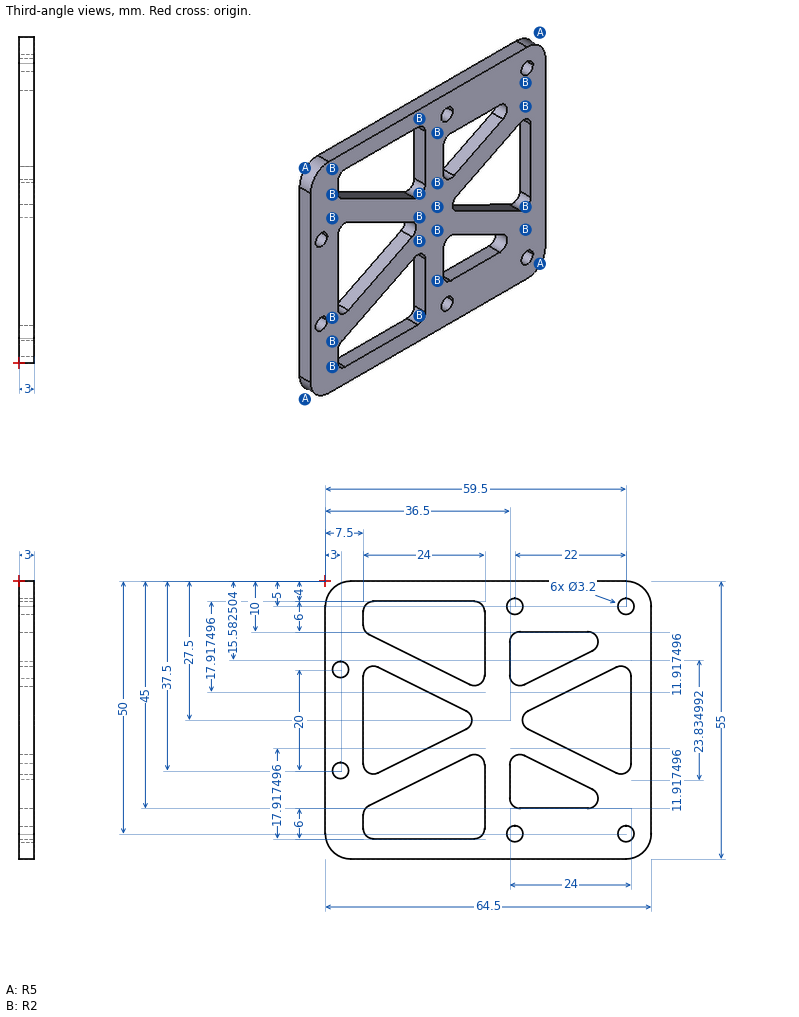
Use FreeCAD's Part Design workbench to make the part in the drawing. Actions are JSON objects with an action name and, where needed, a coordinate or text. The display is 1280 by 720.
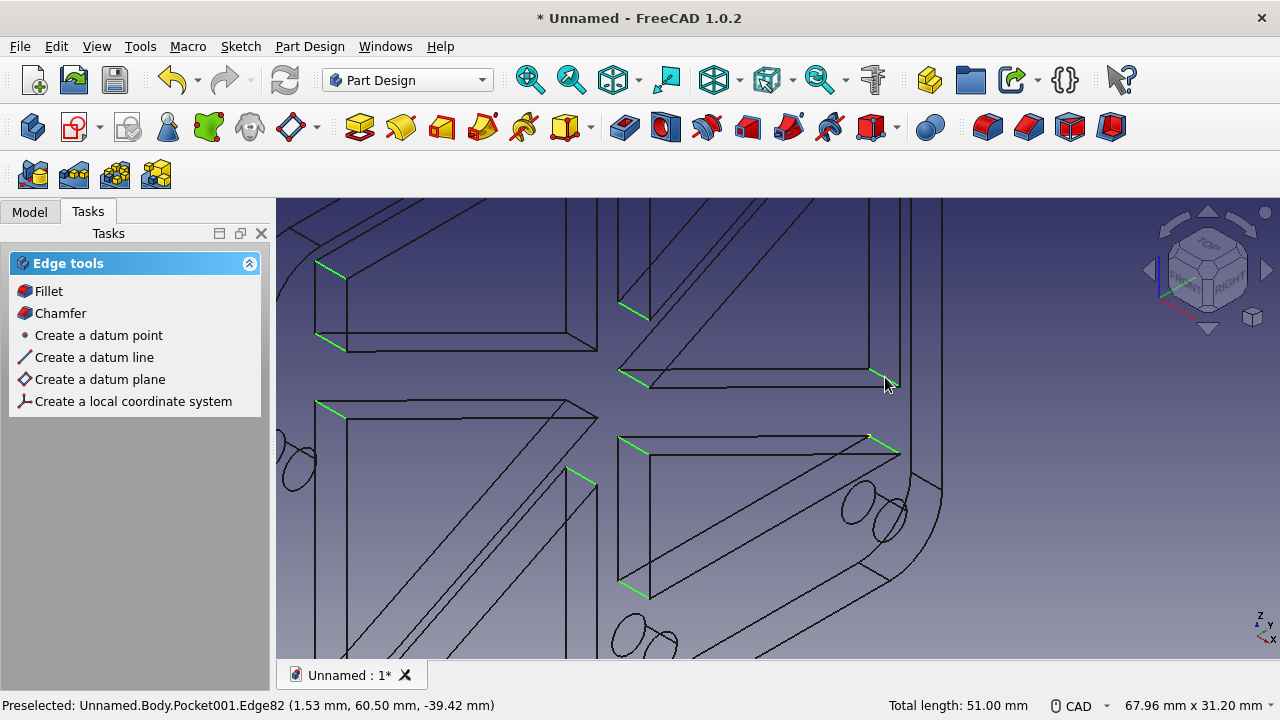
{"action": "left_click", "coordinate": [582, 408], "text": "ctrl"}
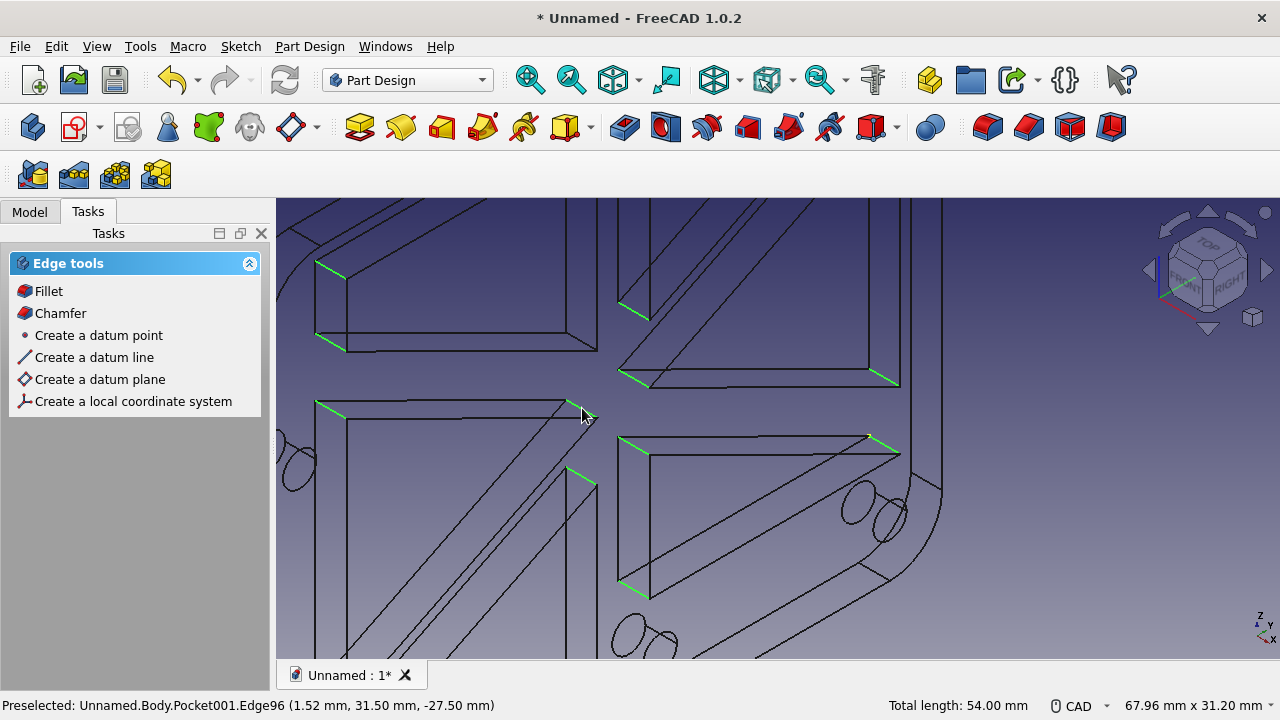
{"action": "left_click", "coordinate": [582, 341], "text": "ctrl"}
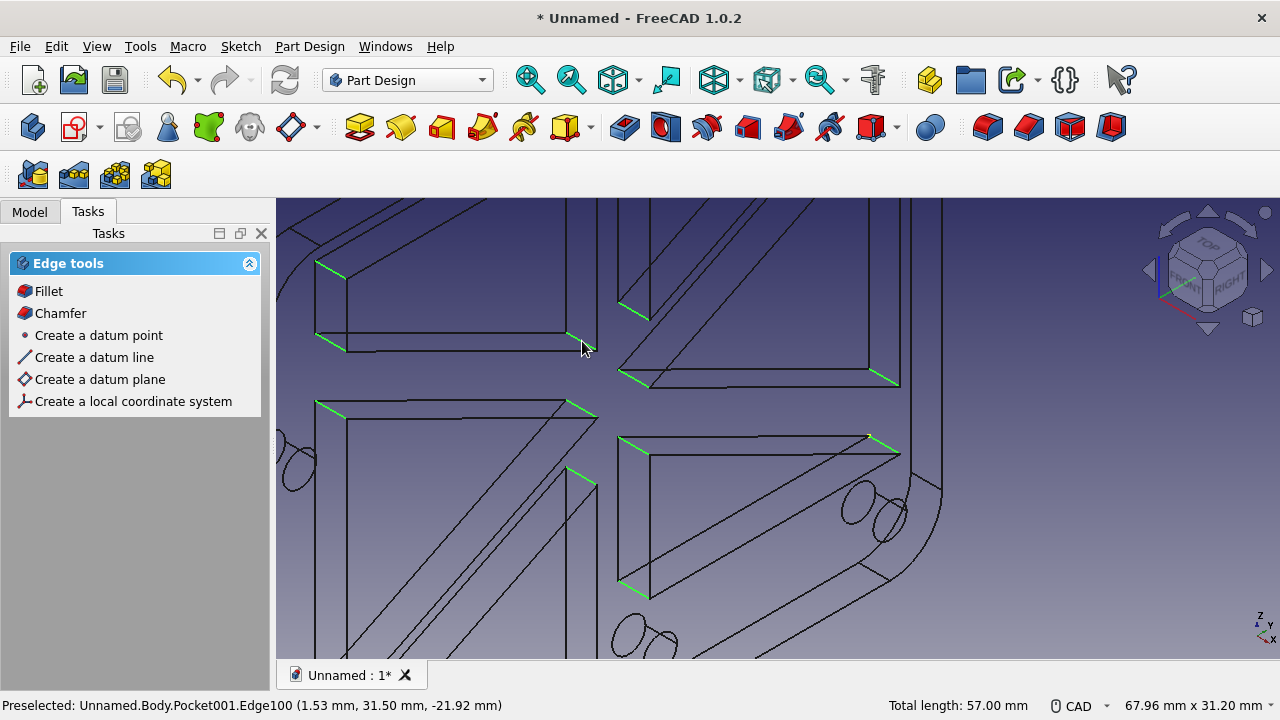
{"action": "key", "text": "v f"}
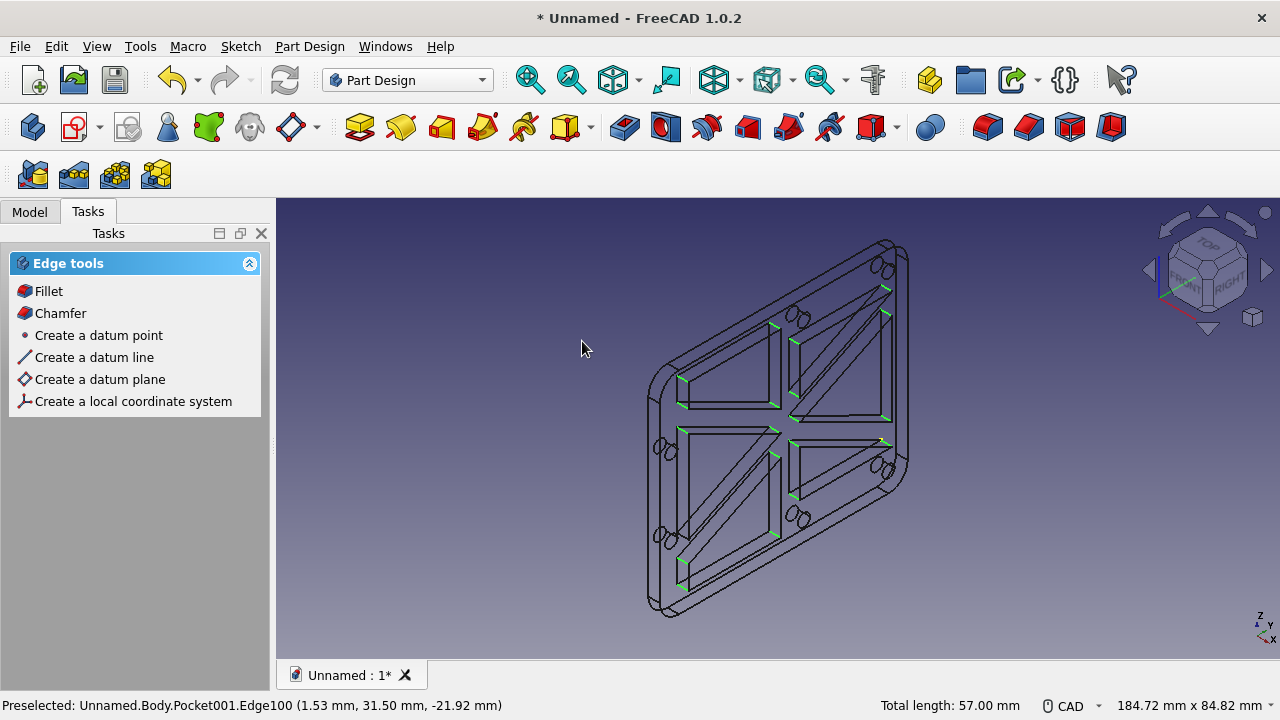
{"action": "key", "text": "2"}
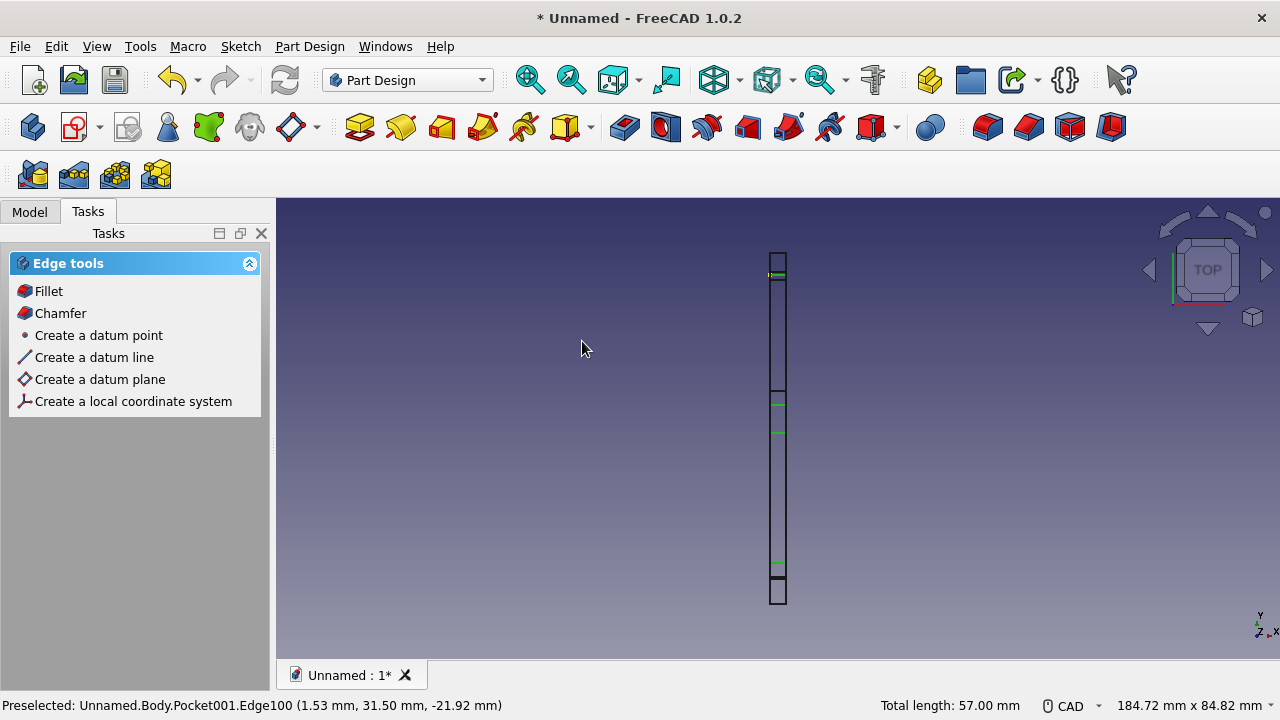
{"action": "scroll", "coordinate": [778, 562], "scroll_direction": "up", "scroll_amount": 5}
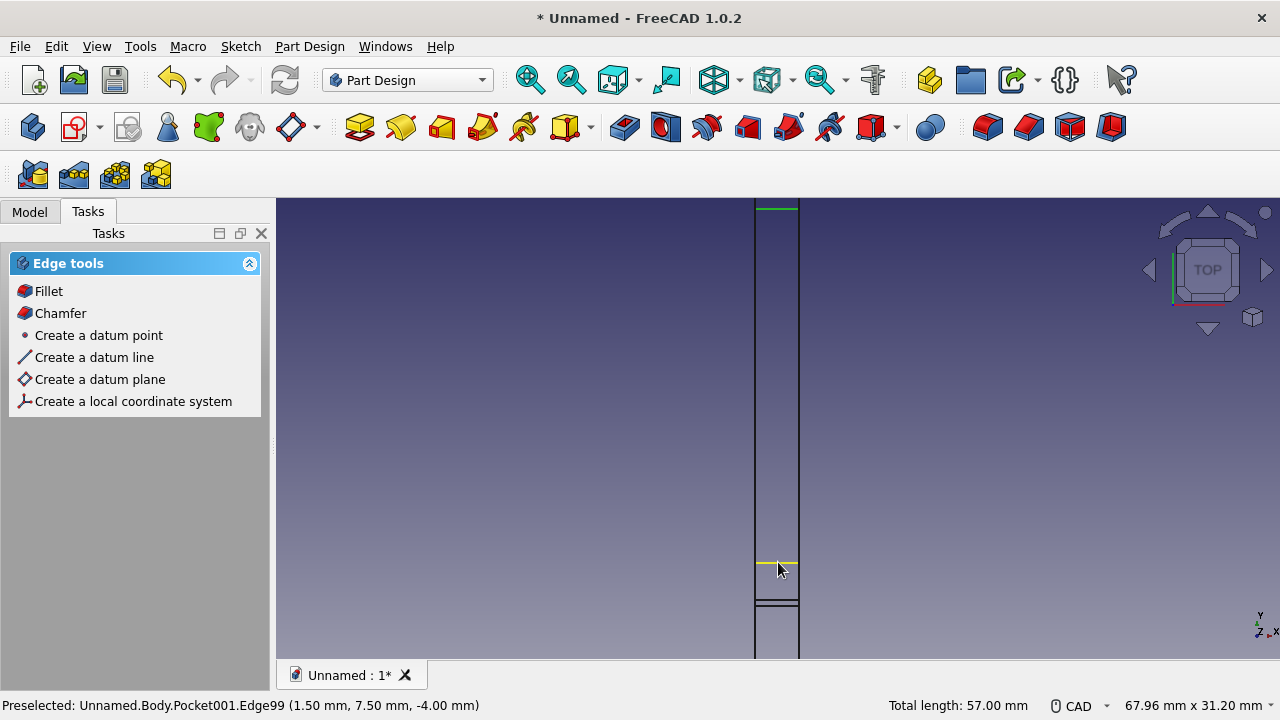
{"action": "left_click", "coordinate": [531, 80]}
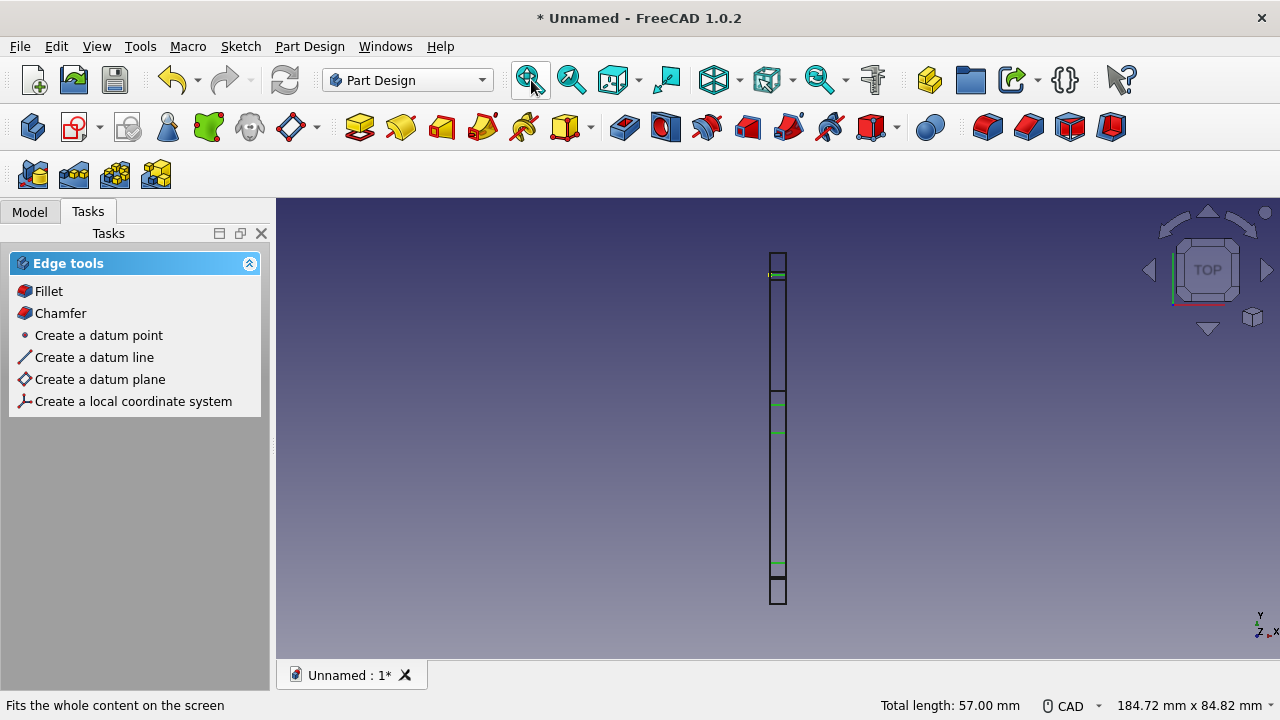
{"action": "key", "text": "1"}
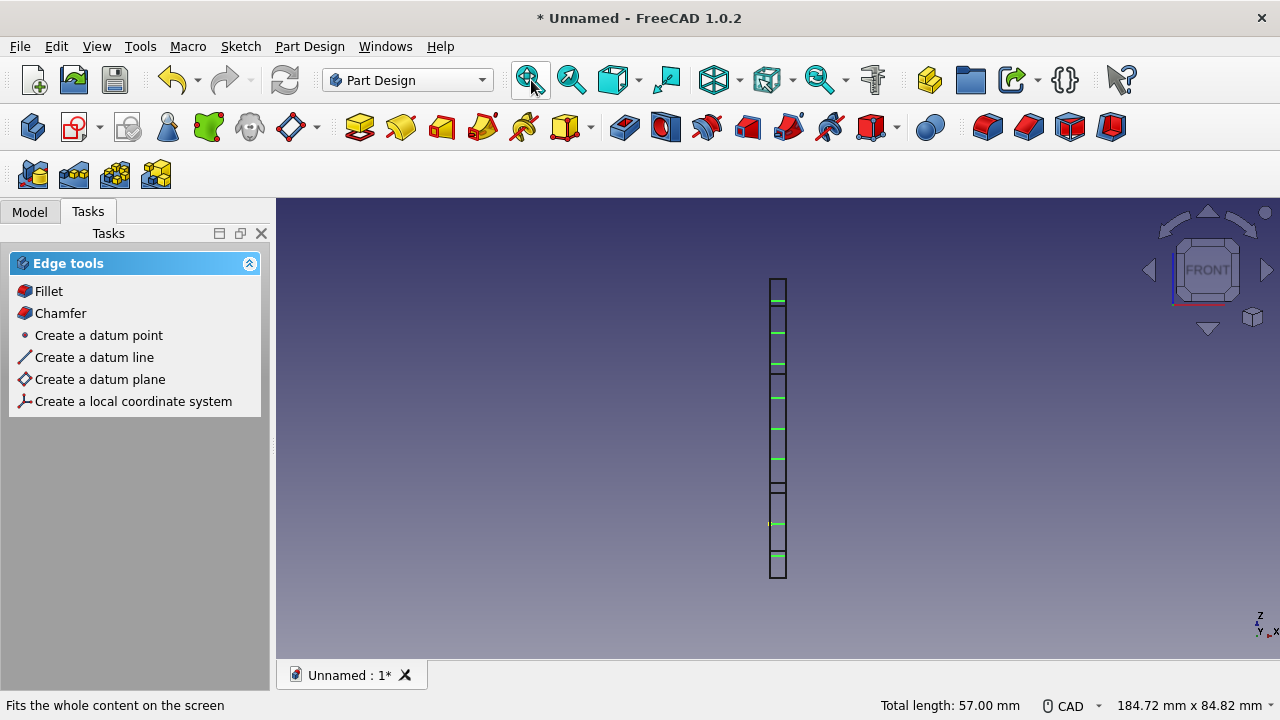
{"action": "left_click", "coordinate": [778, 492], "text": "ctrl"}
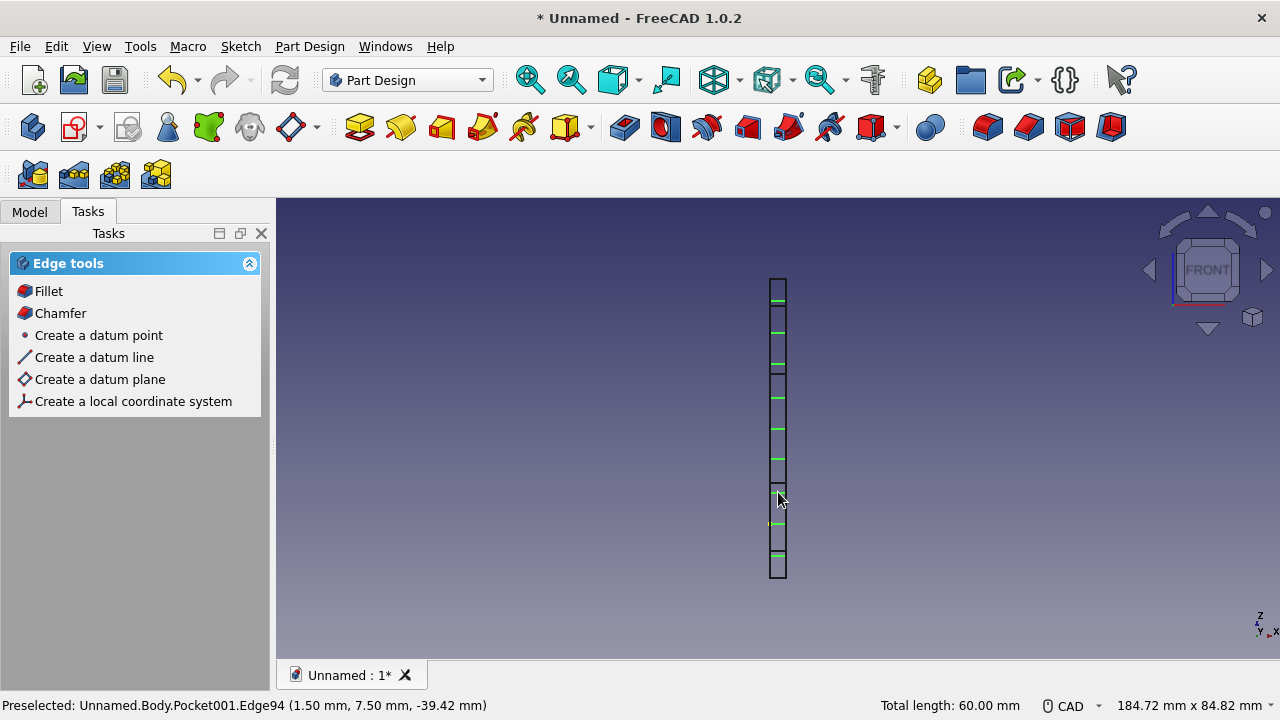
{"action": "key", "text": "v 1"}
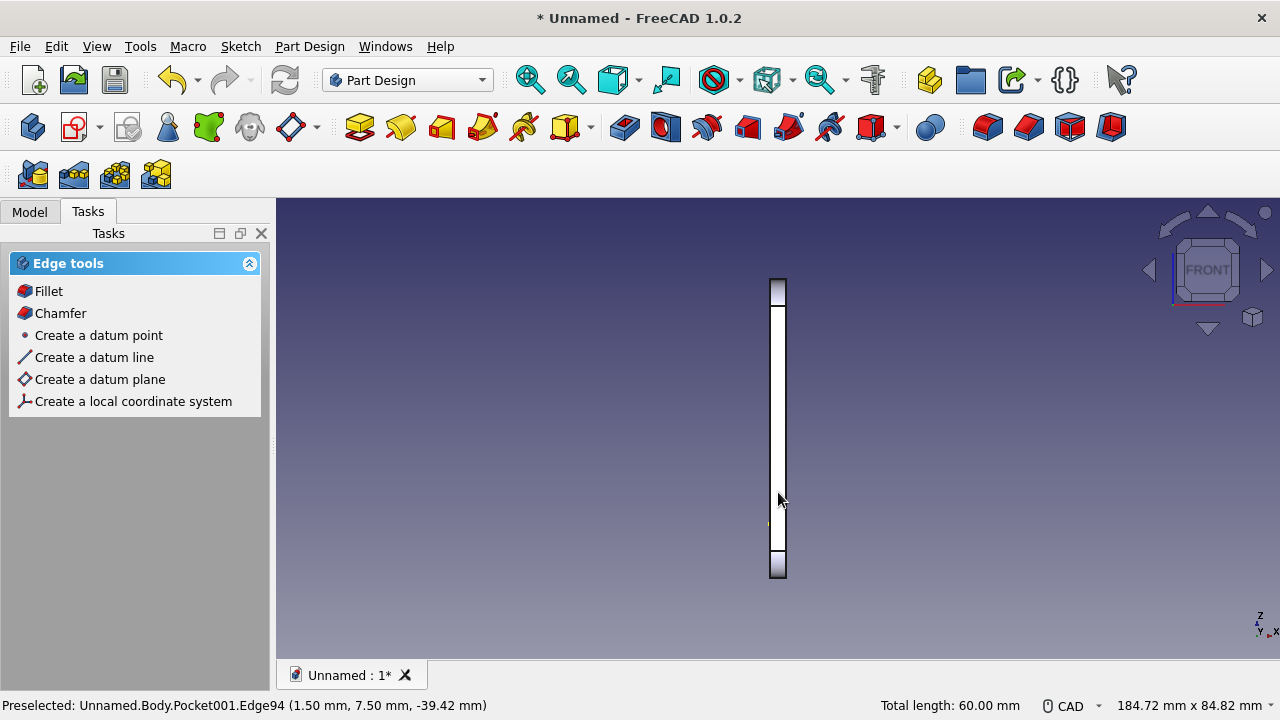
{"action": "left_click", "coordinate": [988, 128]}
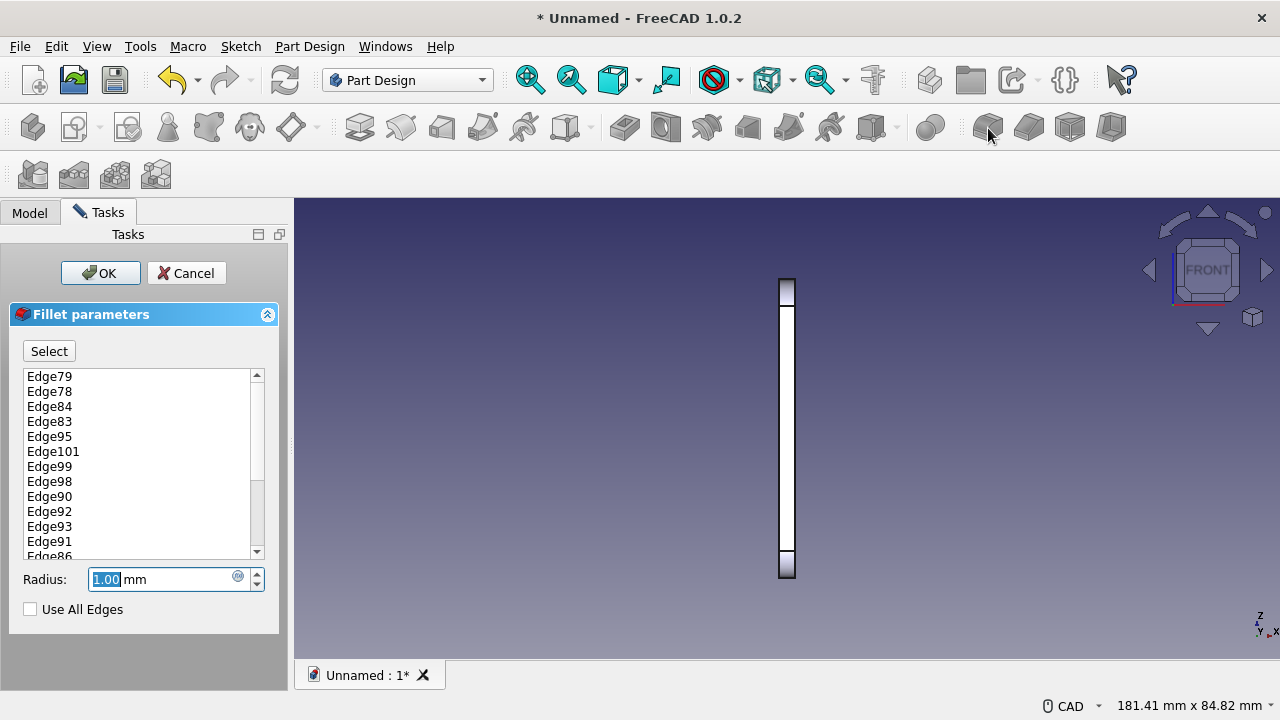
{"action": "type", "text": "2"}
{"action": "key", "text": "Tab"}